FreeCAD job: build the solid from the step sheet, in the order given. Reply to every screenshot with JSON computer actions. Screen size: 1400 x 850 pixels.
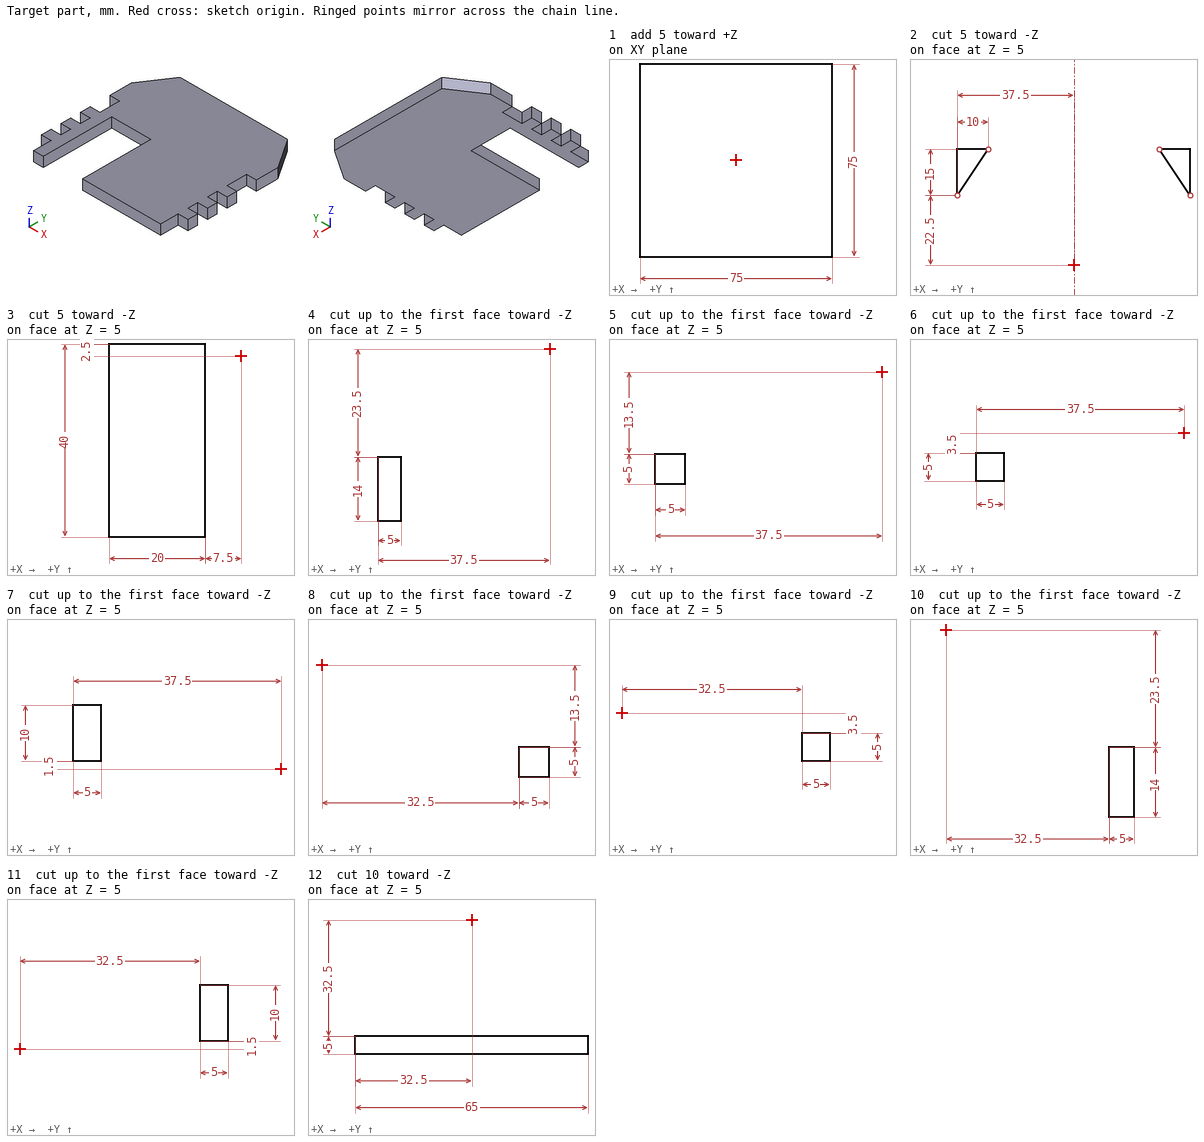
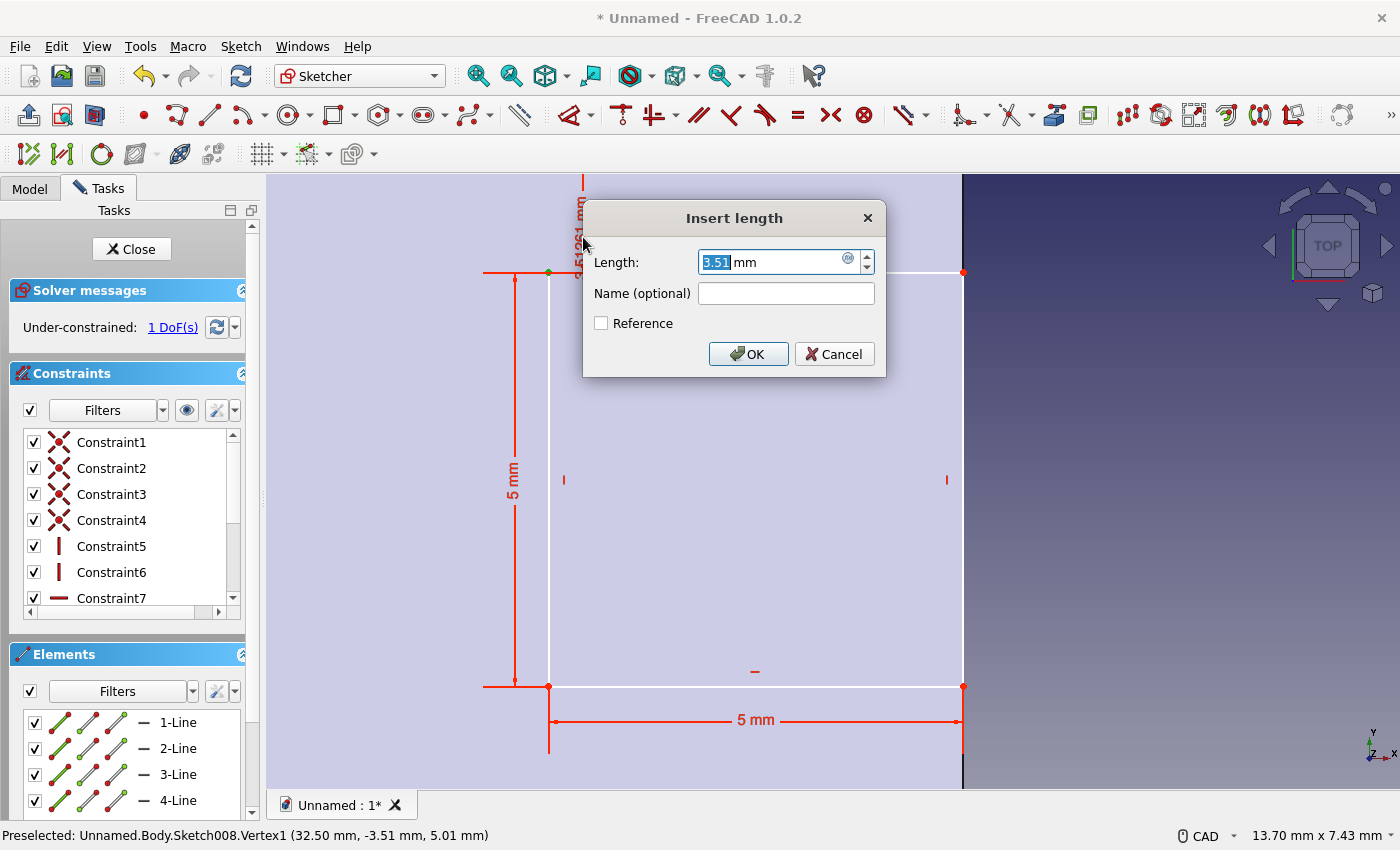
{"action": "type", "text": "3.5"}
{"action": "key", "text": "Return"}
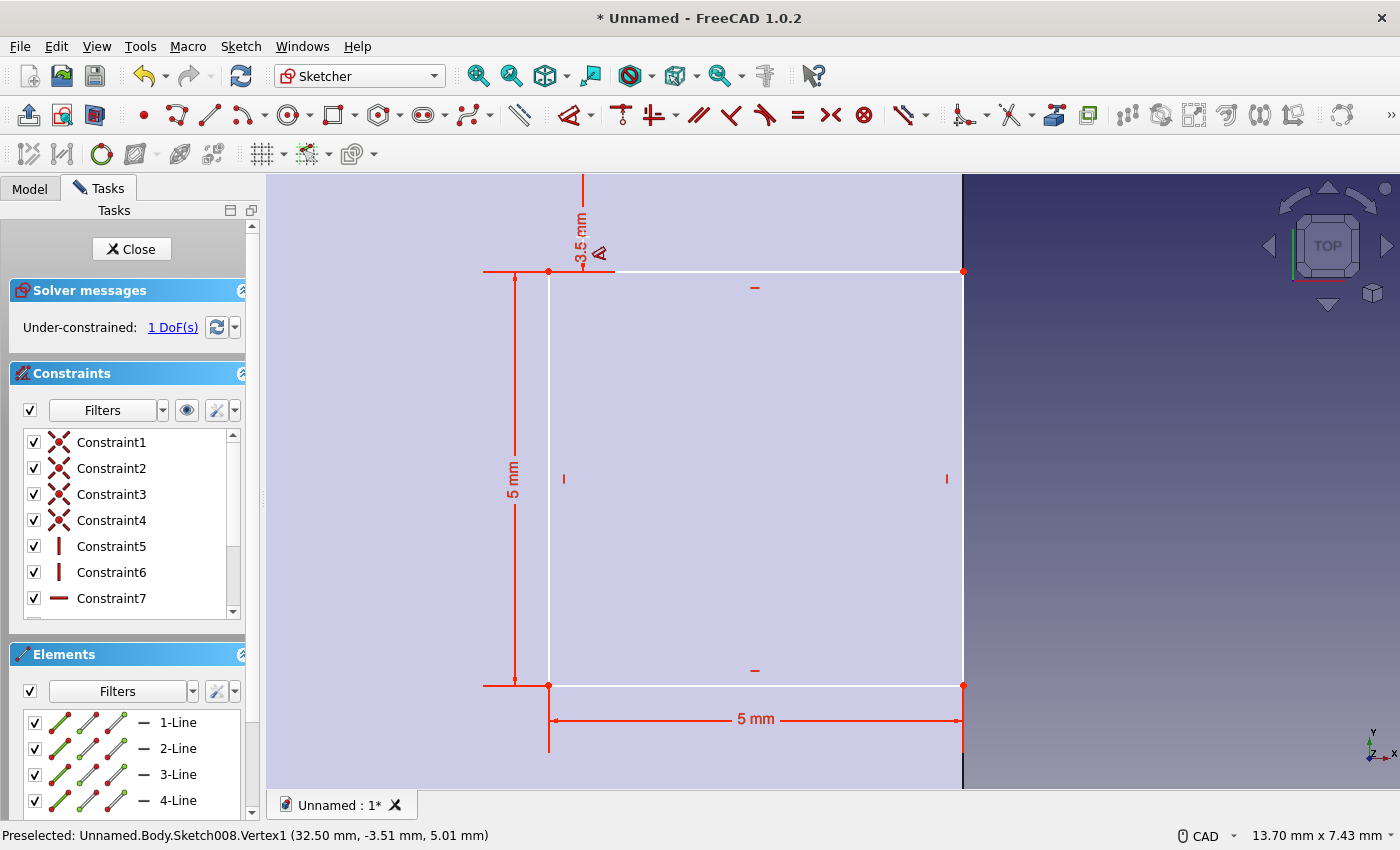
{"action": "left_click", "coordinate": [549, 272]}
{"action": "left_click", "coordinate": [421, 306]}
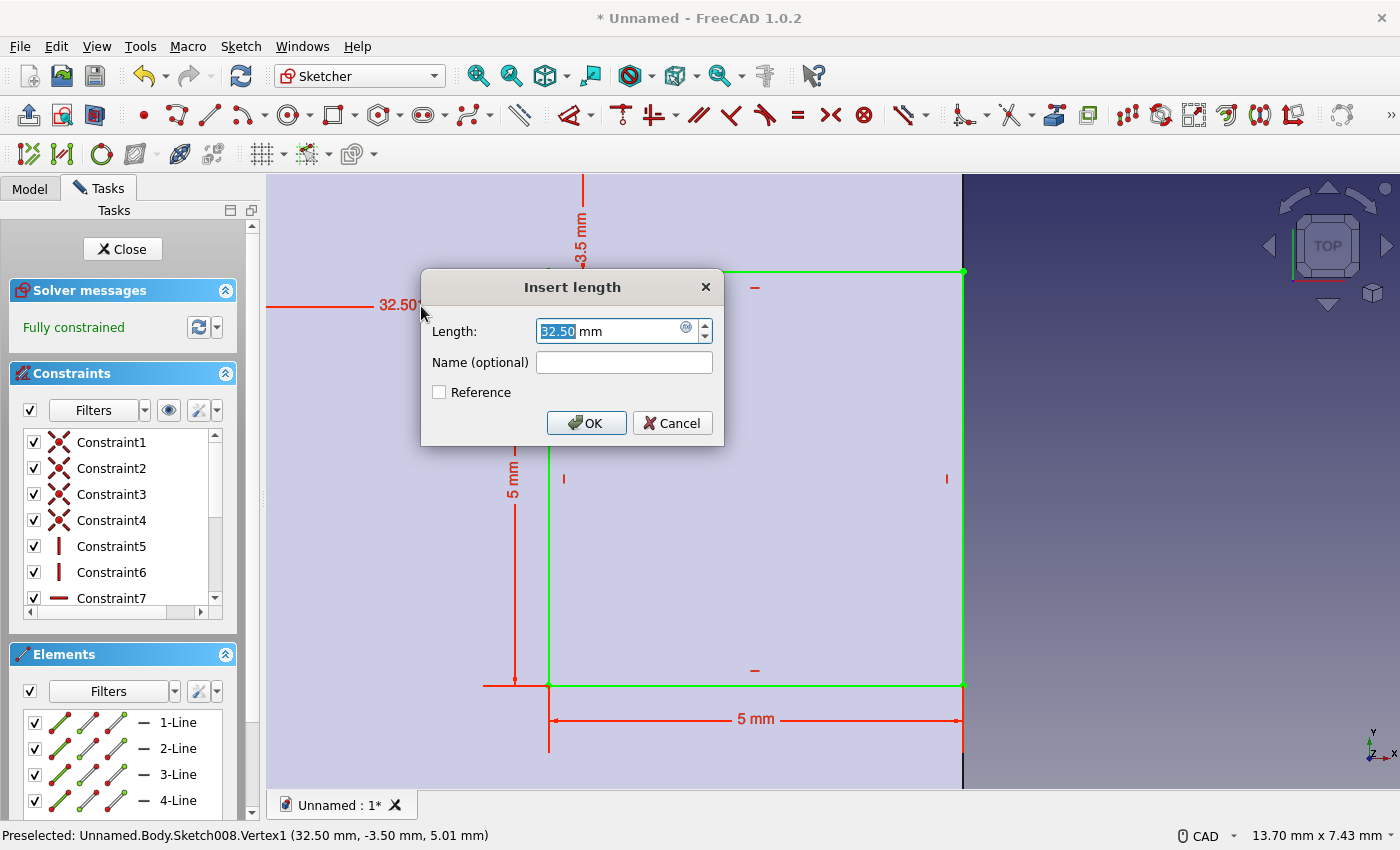
{"action": "type", "text": "32.5"}
{"action": "key", "text": "Return"}
{"action": "key", "text": "Escape"}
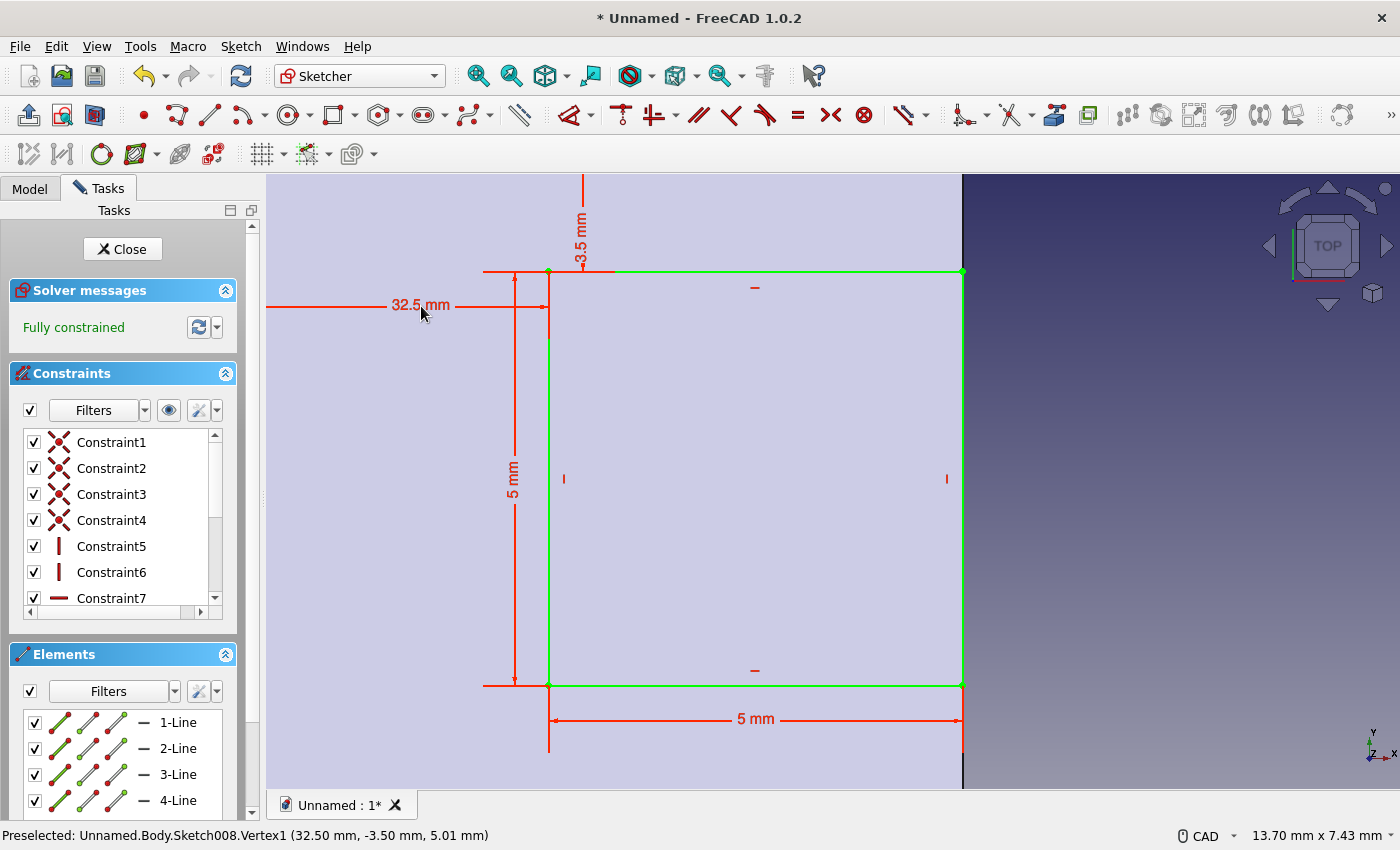
{"action": "left_click", "coordinate": [123, 249]}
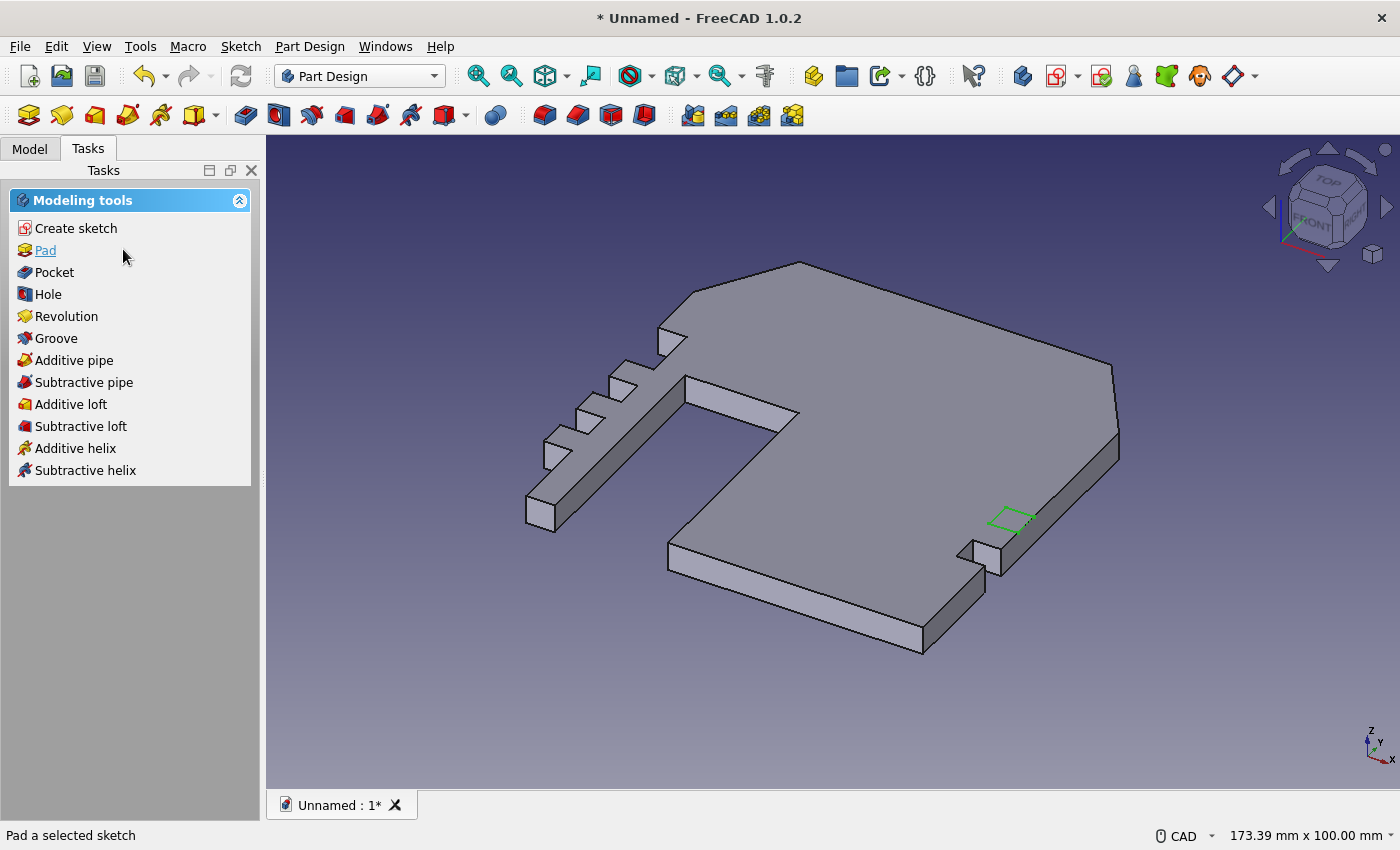
{"action": "left_click", "coordinate": [246, 116]}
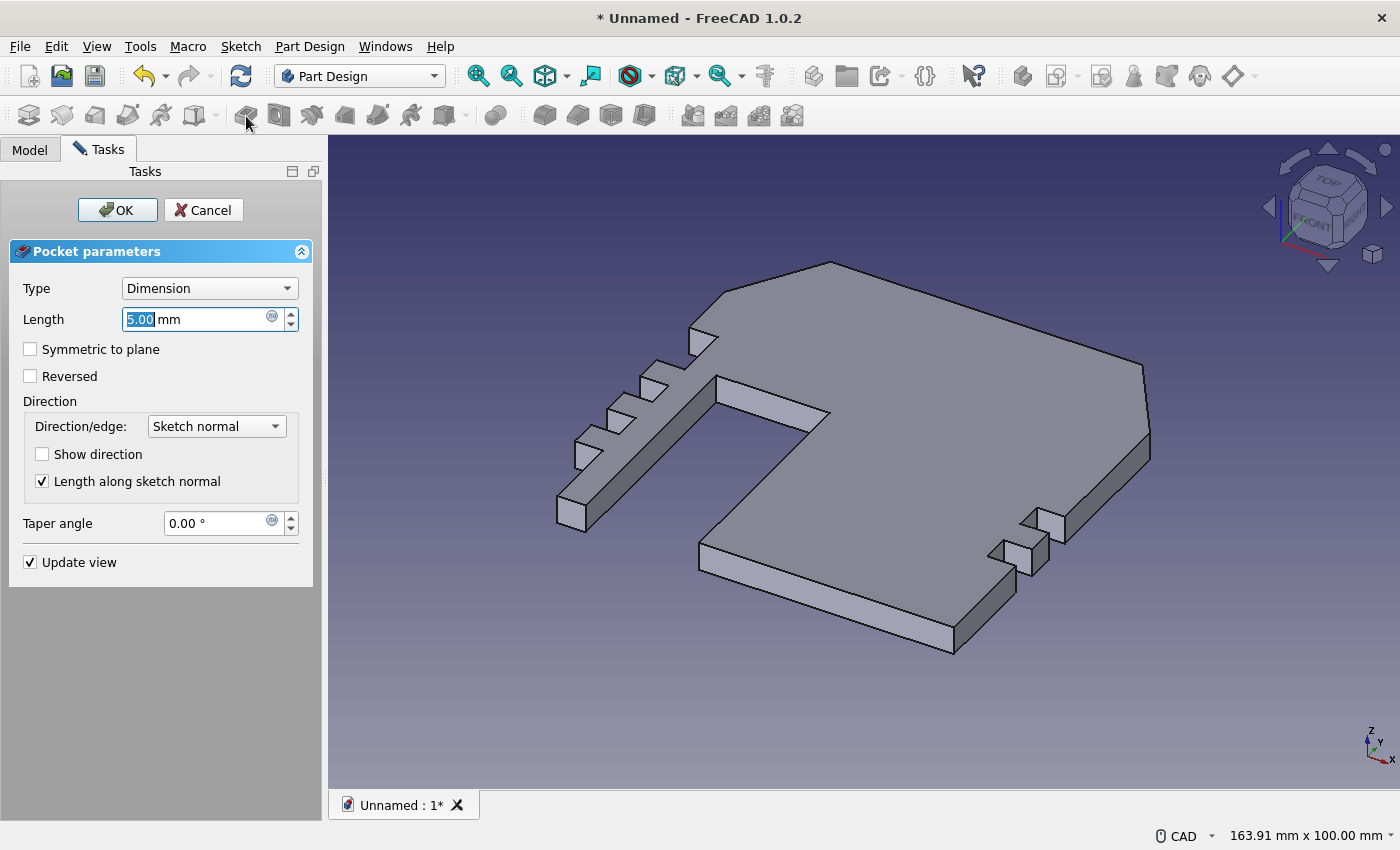
{"action": "left_click", "coordinate": [210, 288]}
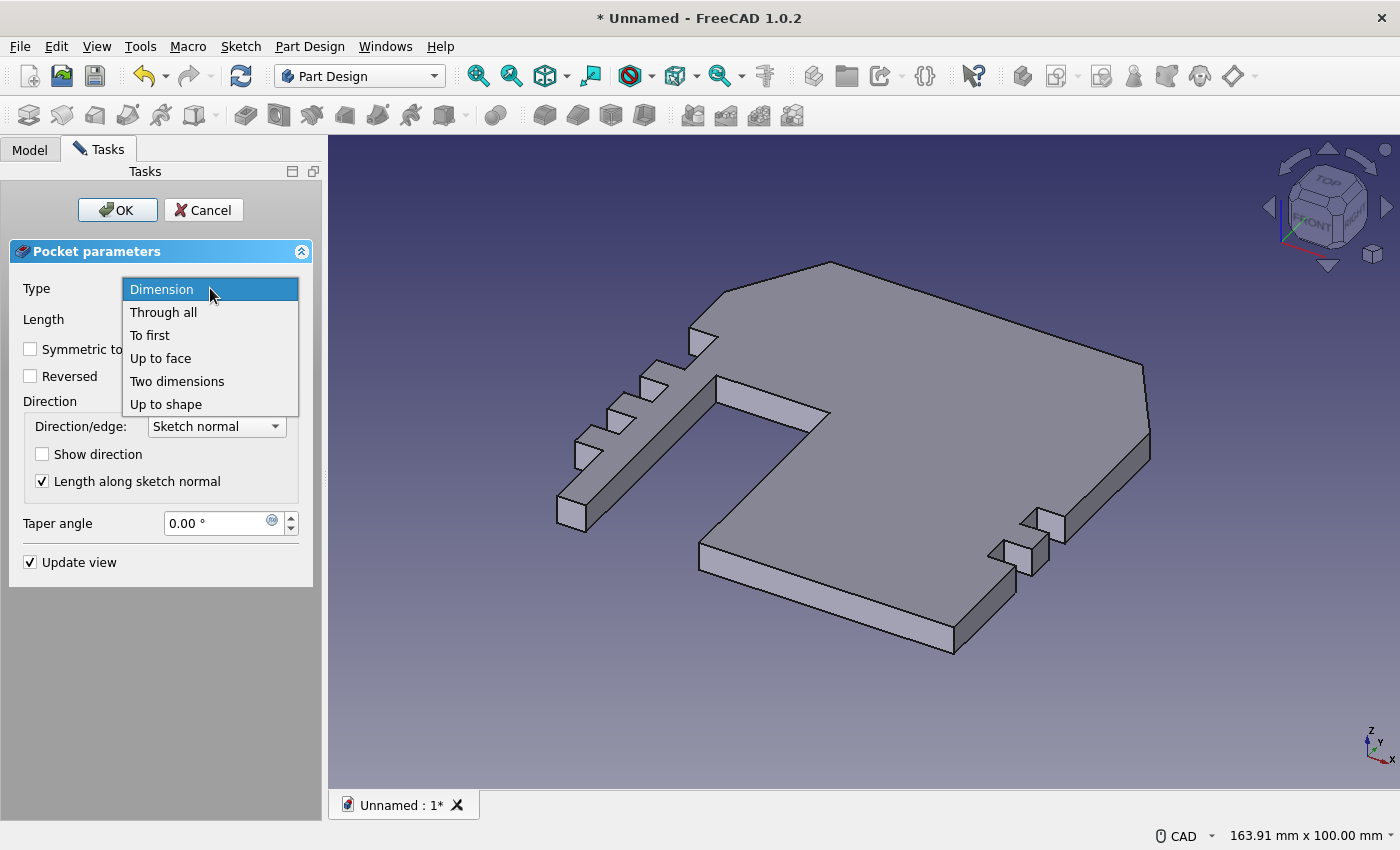
{"action": "left_click", "coordinate": [208, 336]}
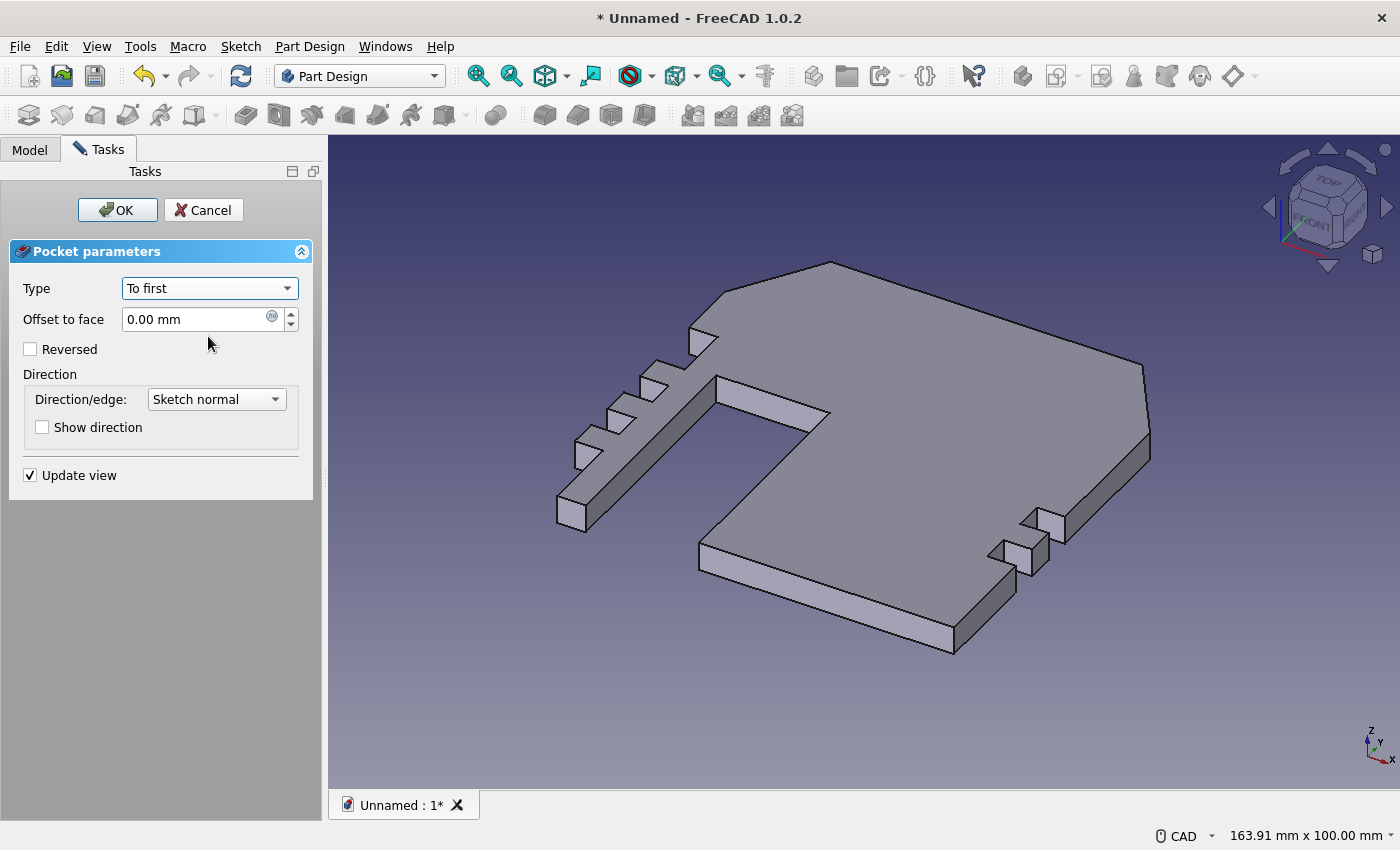
{"action": "left_click", "coordinate": [118, 210]}